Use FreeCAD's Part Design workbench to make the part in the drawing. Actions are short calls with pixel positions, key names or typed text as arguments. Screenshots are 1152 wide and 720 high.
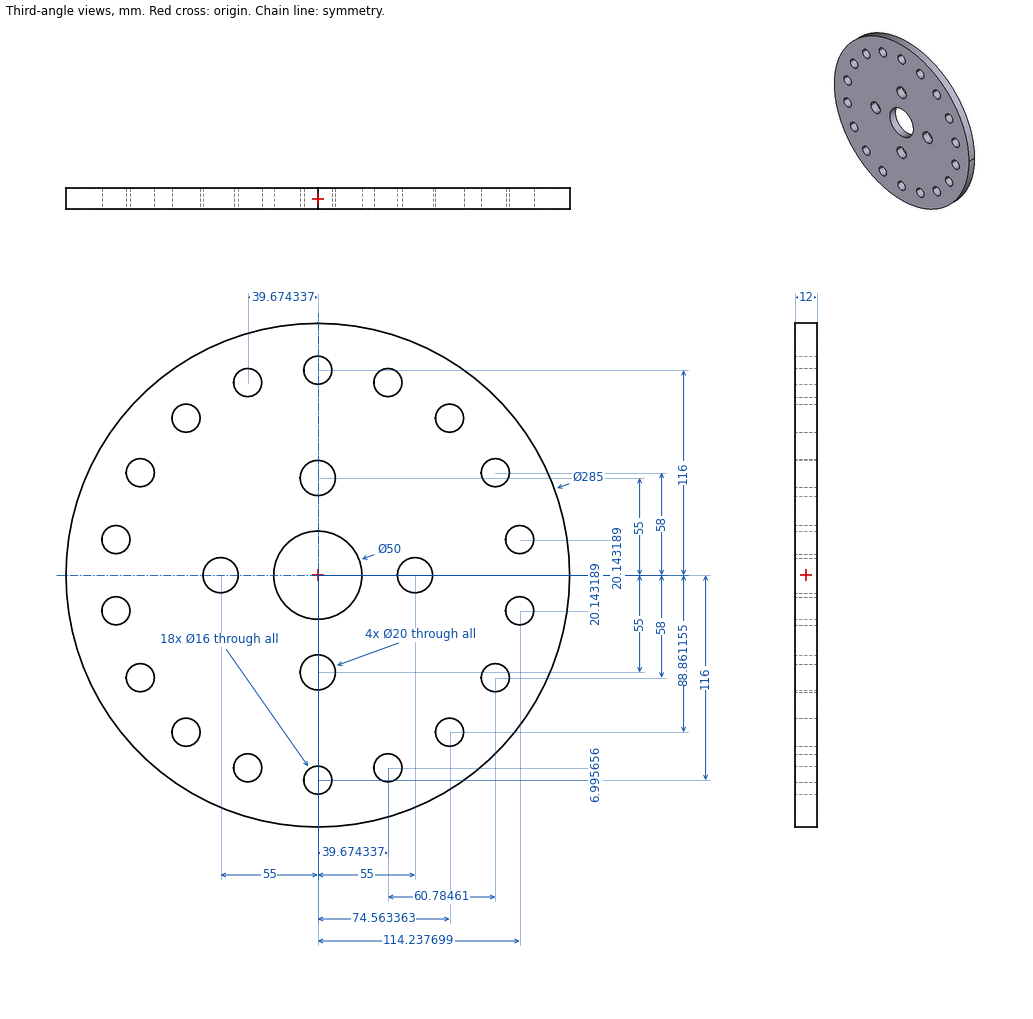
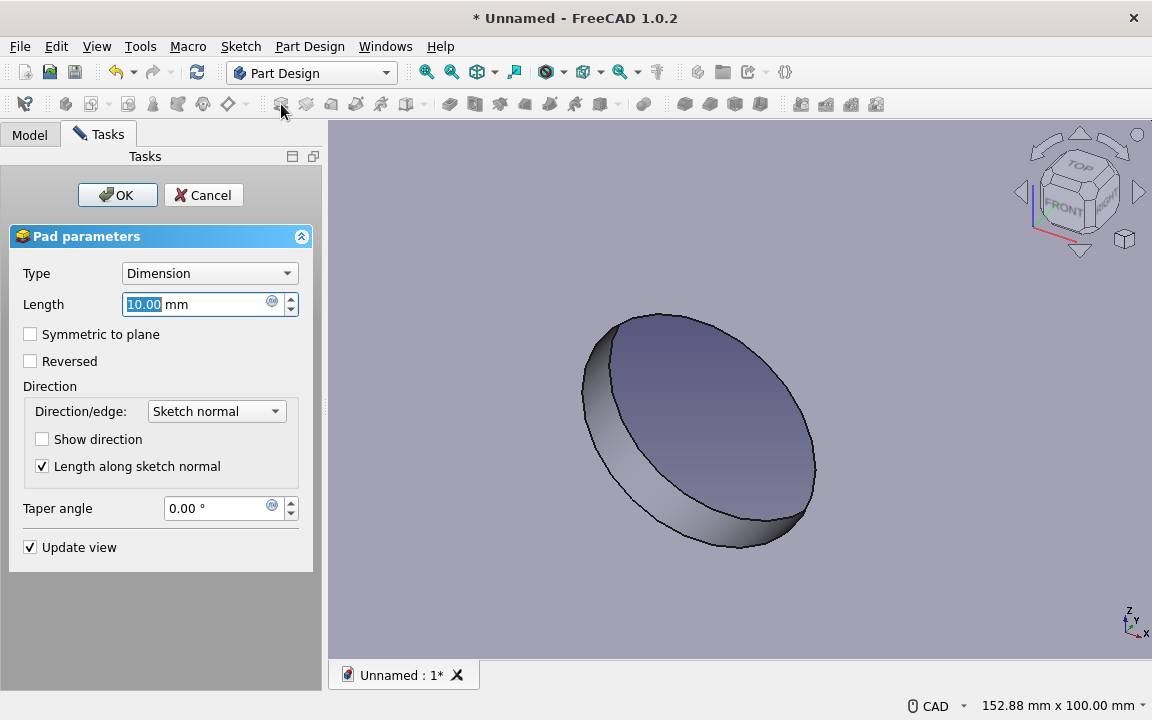
text(12)
key(Tab)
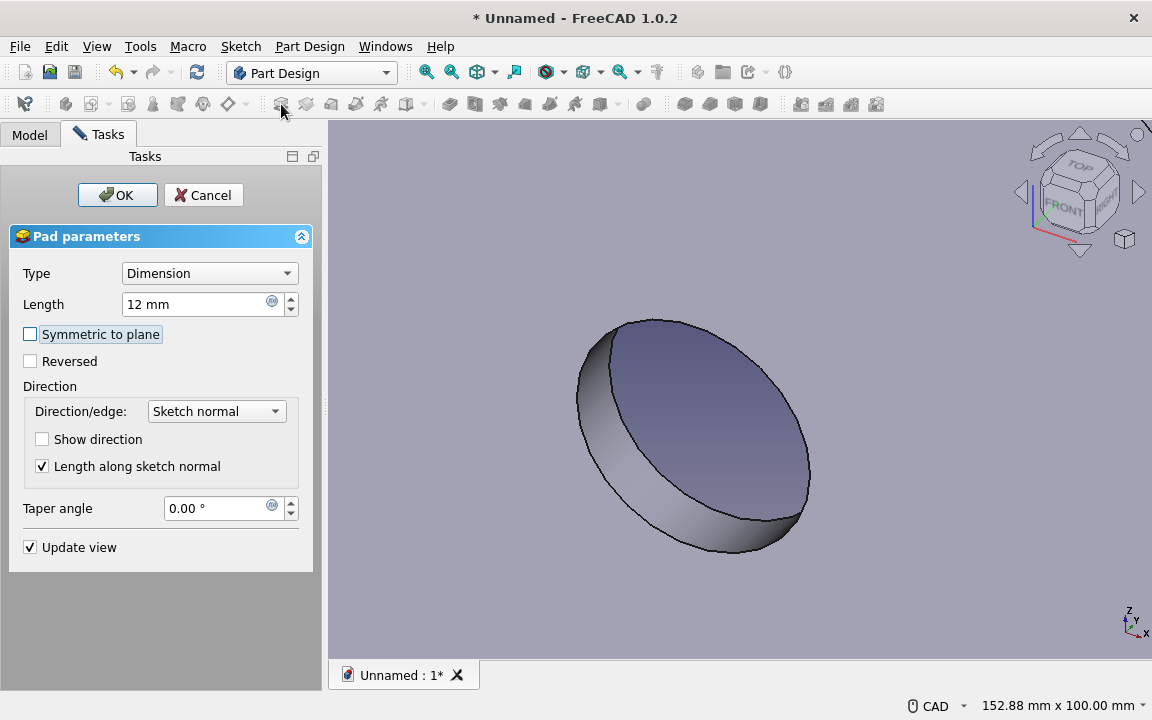
click(31, 334)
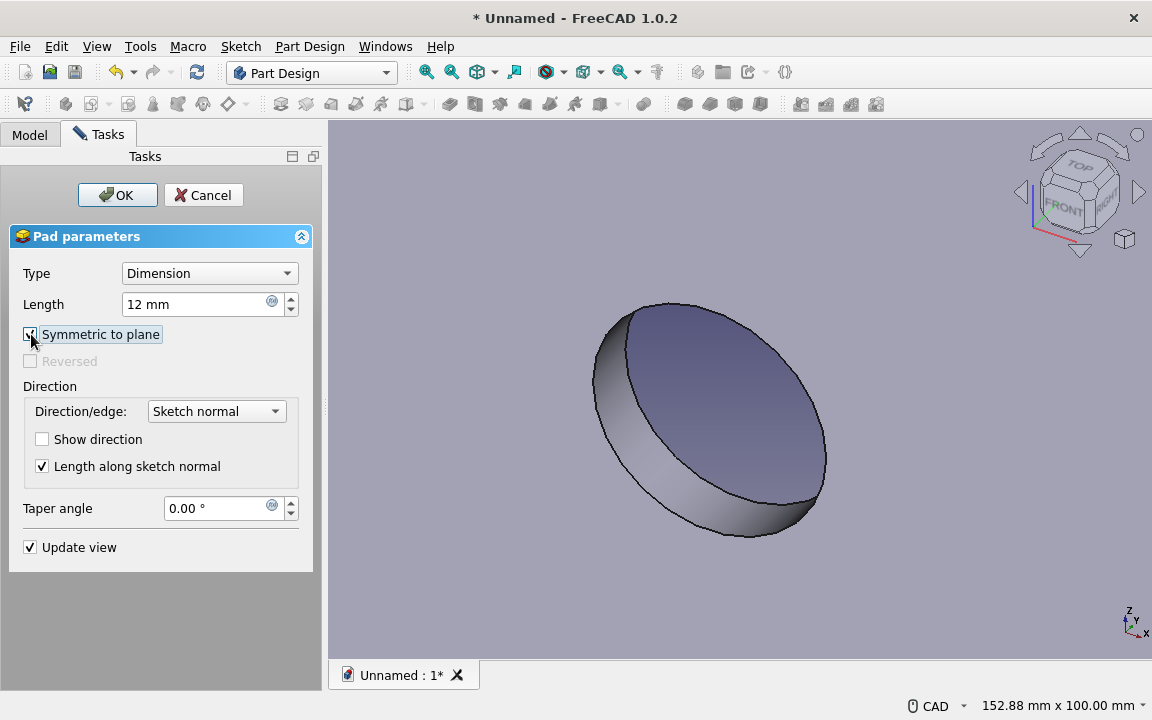
click(118, 195)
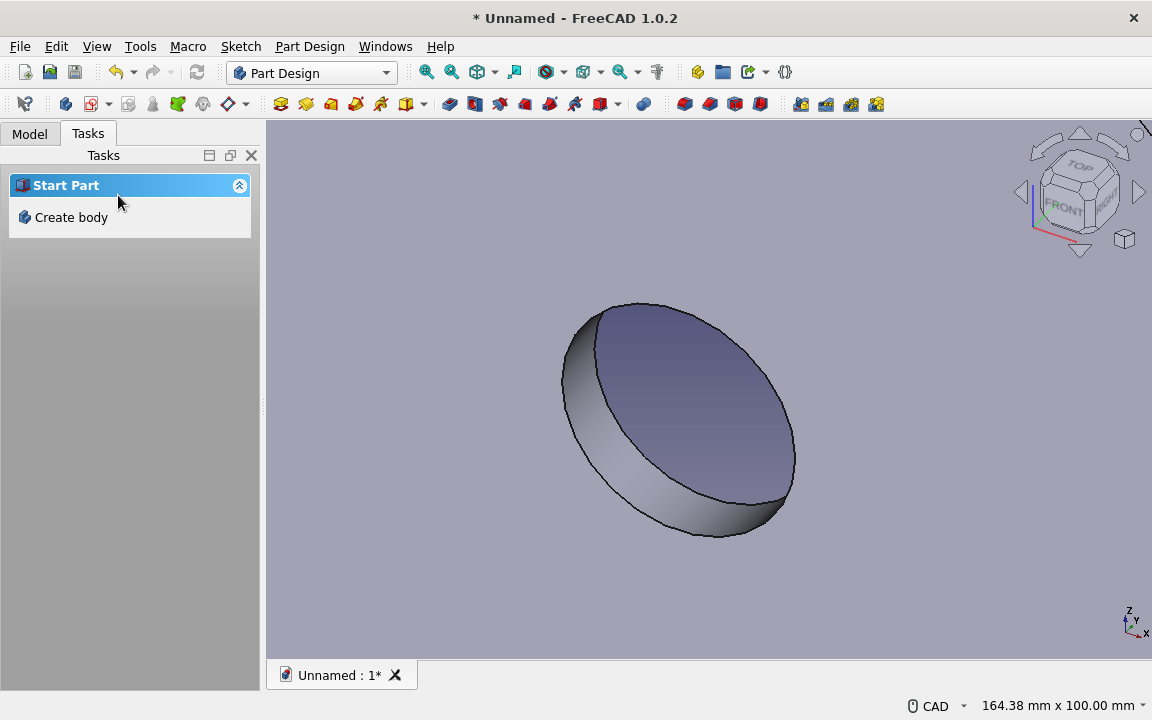
click(427, 72)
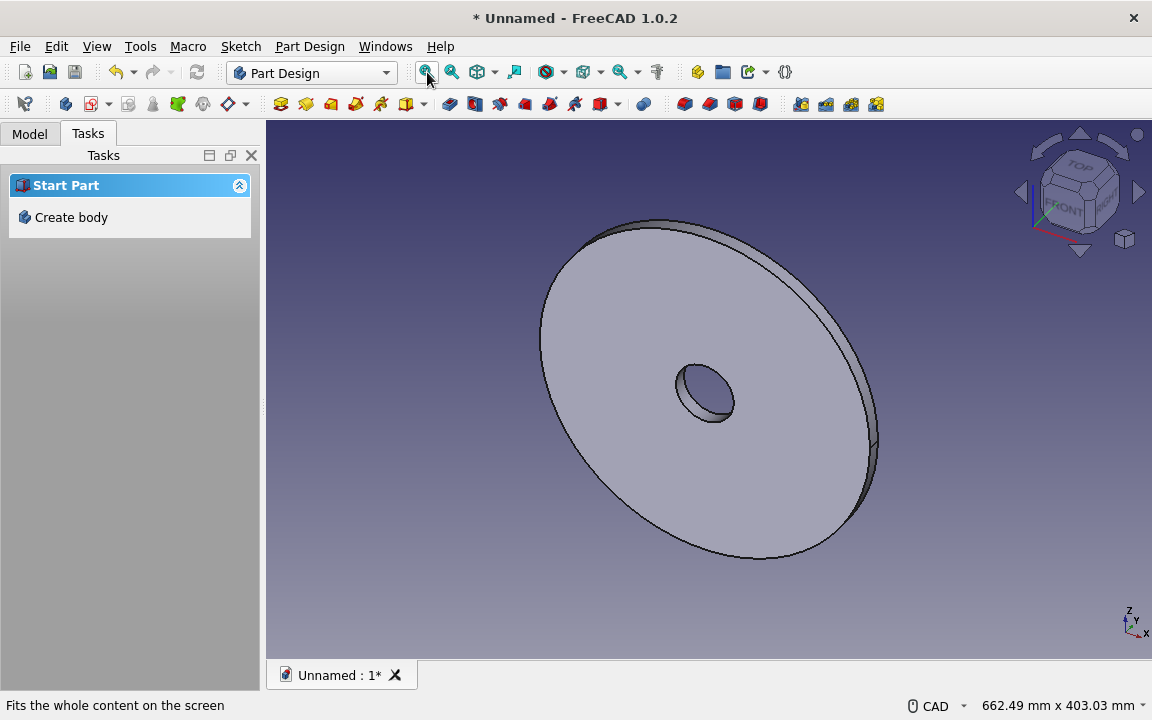
key(4)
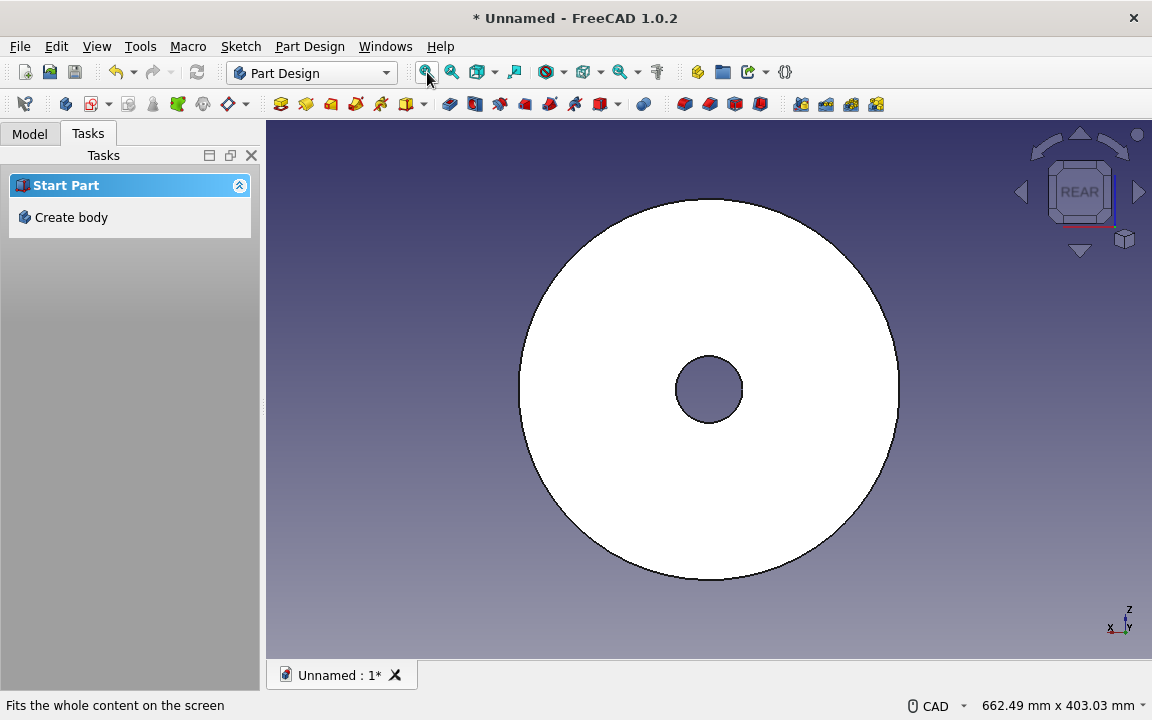
click(709, 497)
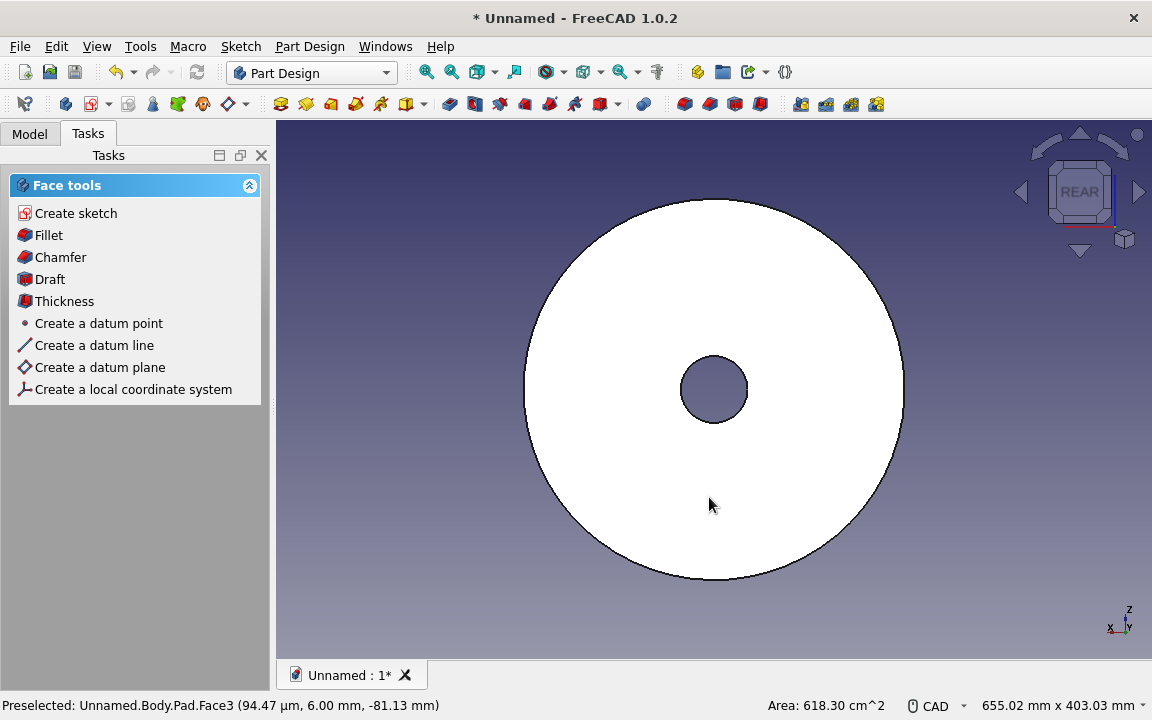
click(90, 104)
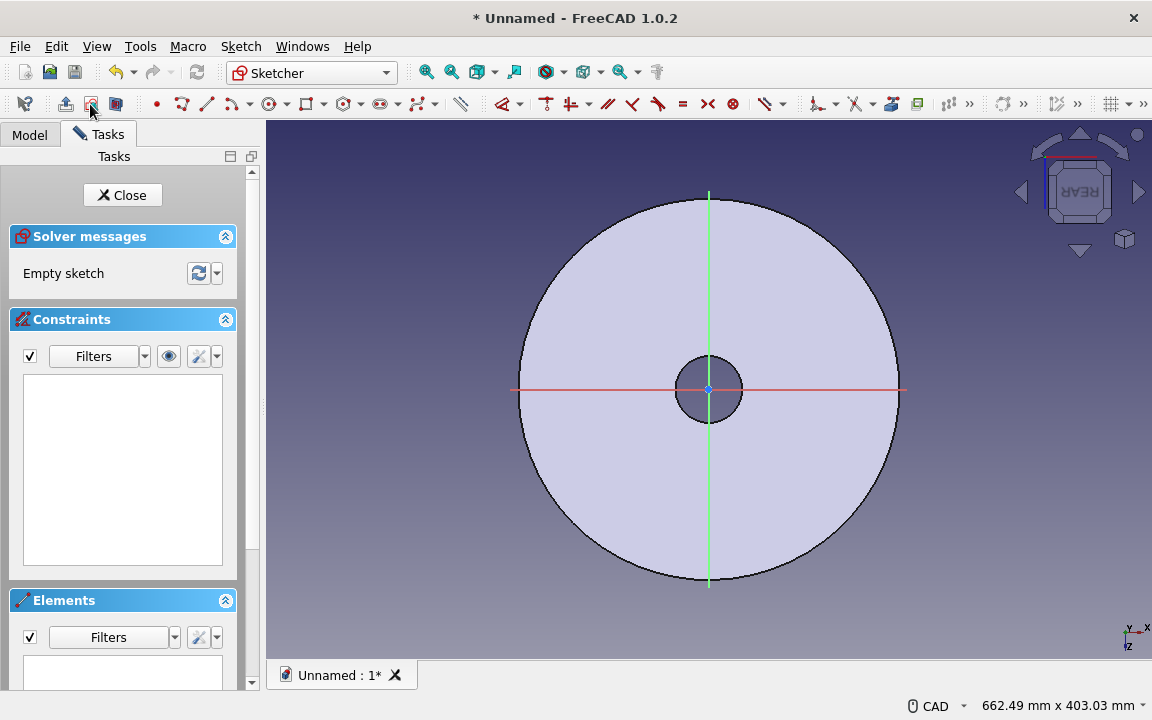
scroll(792, 390, up, 3)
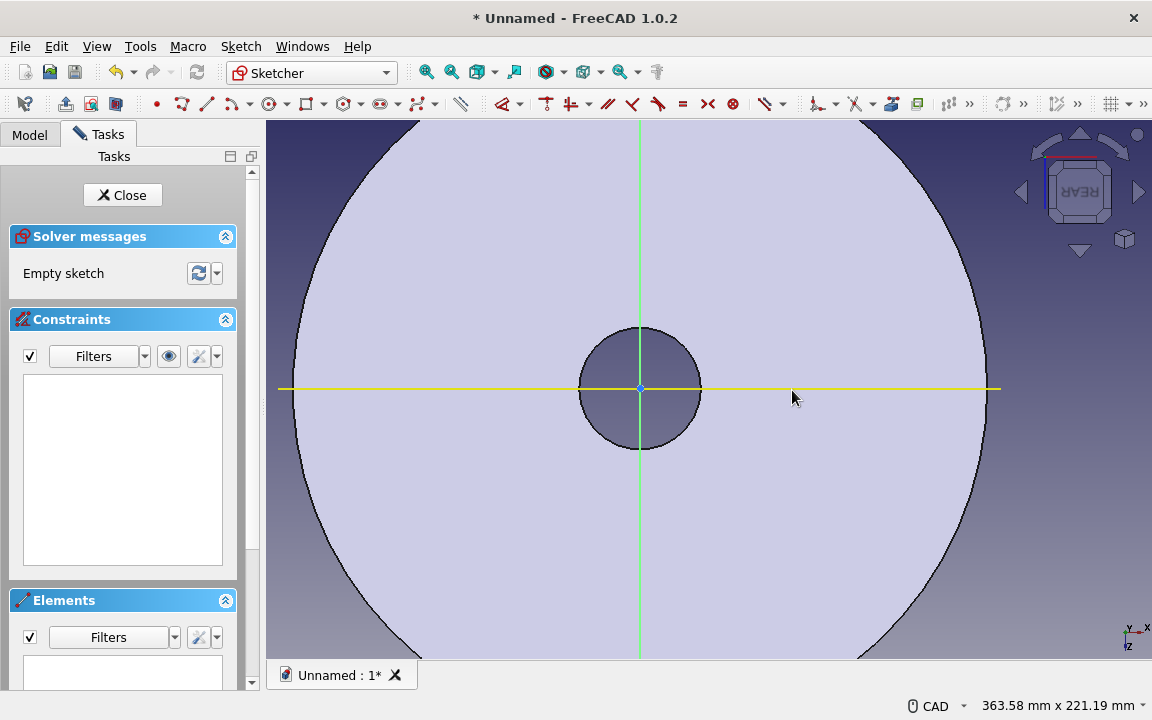
click(268, 104)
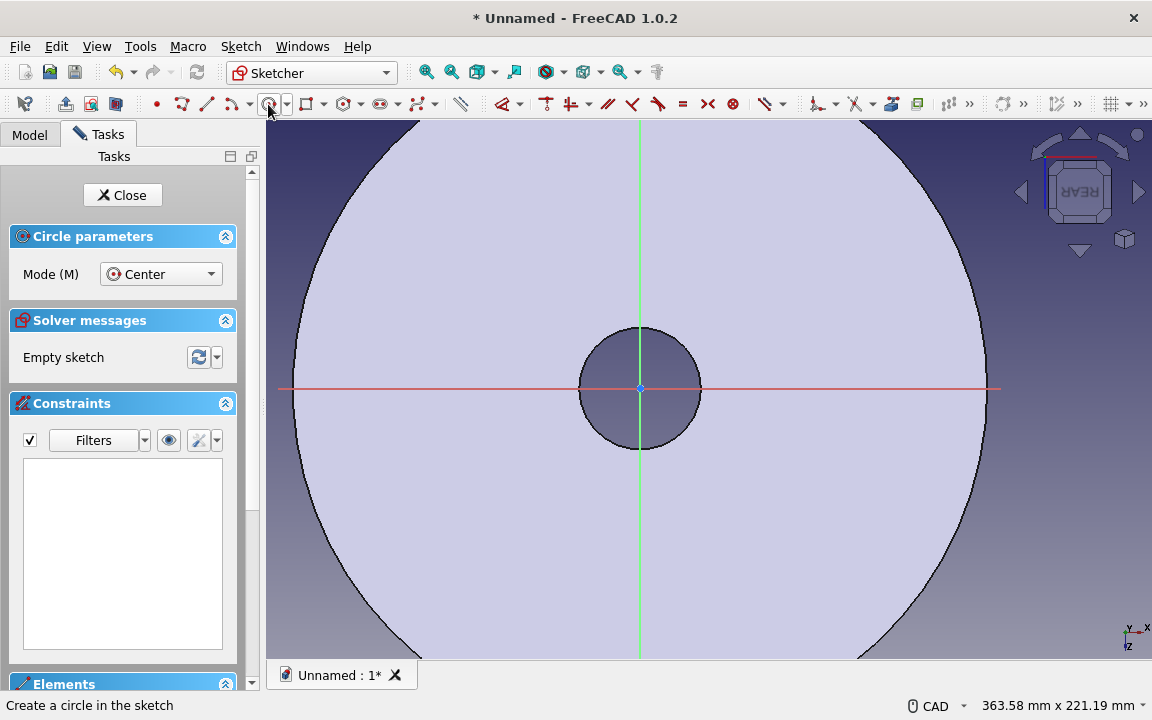
click(640, 255)
move(657, 237)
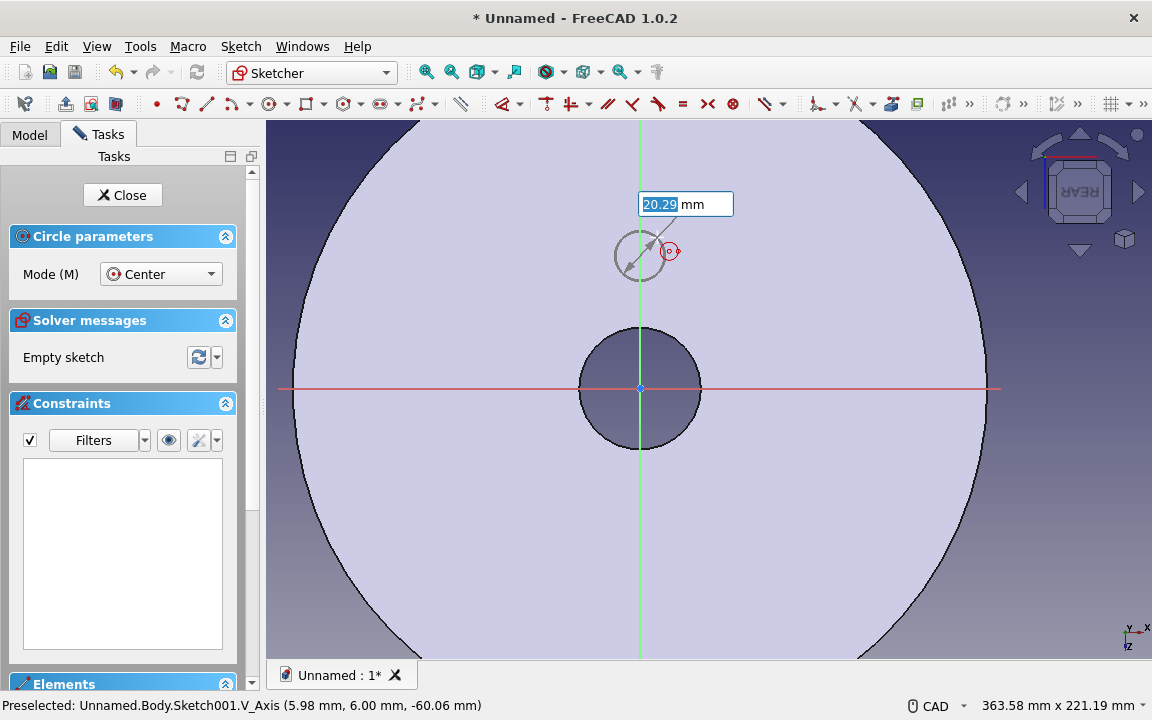
text(20)
key(Return)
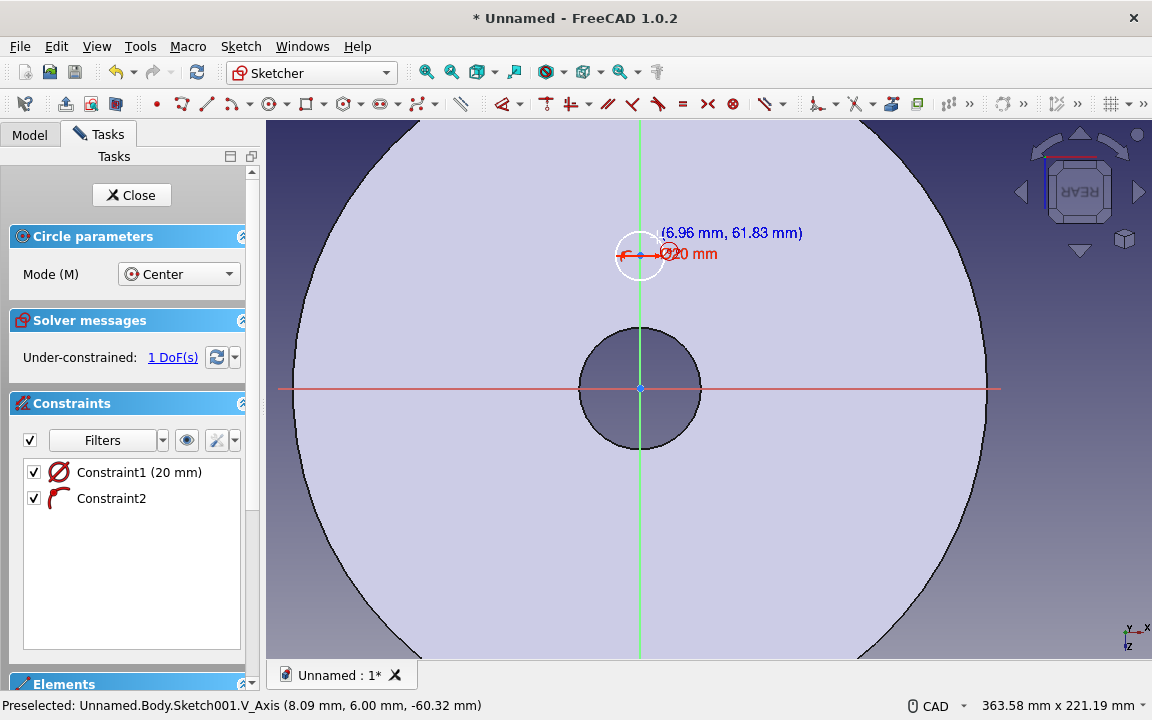
click(774, 389)
move(791, 371)